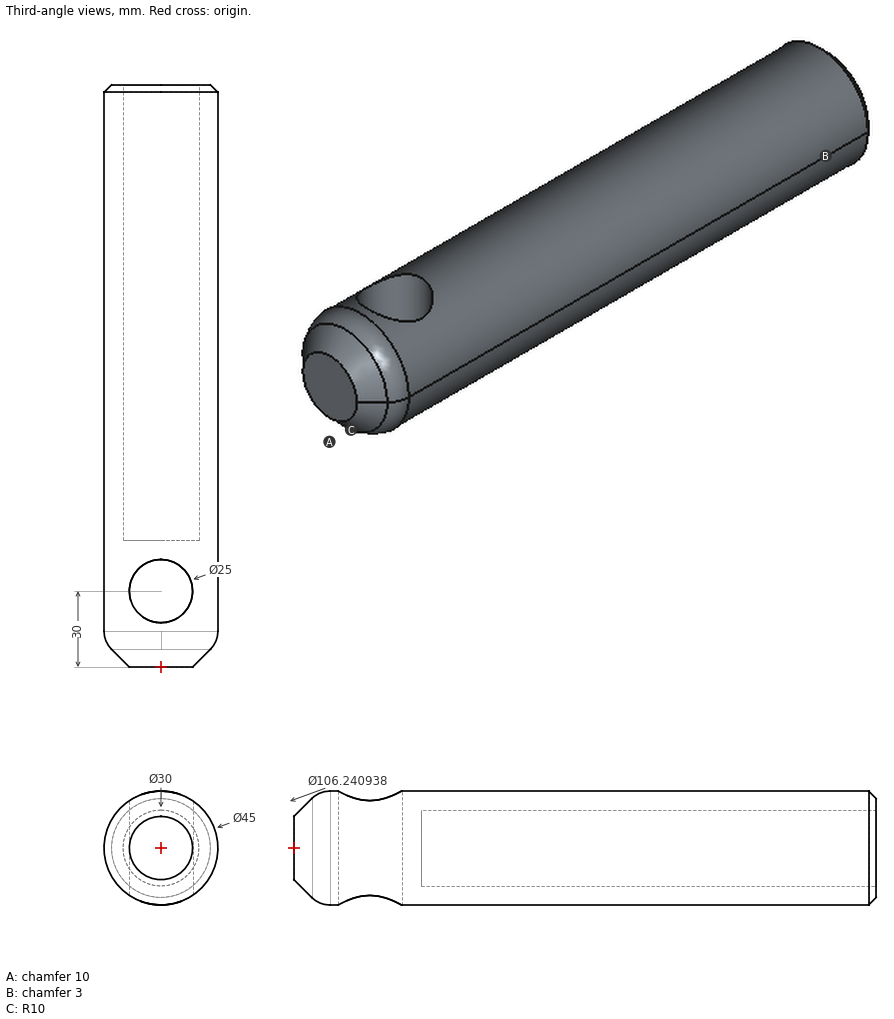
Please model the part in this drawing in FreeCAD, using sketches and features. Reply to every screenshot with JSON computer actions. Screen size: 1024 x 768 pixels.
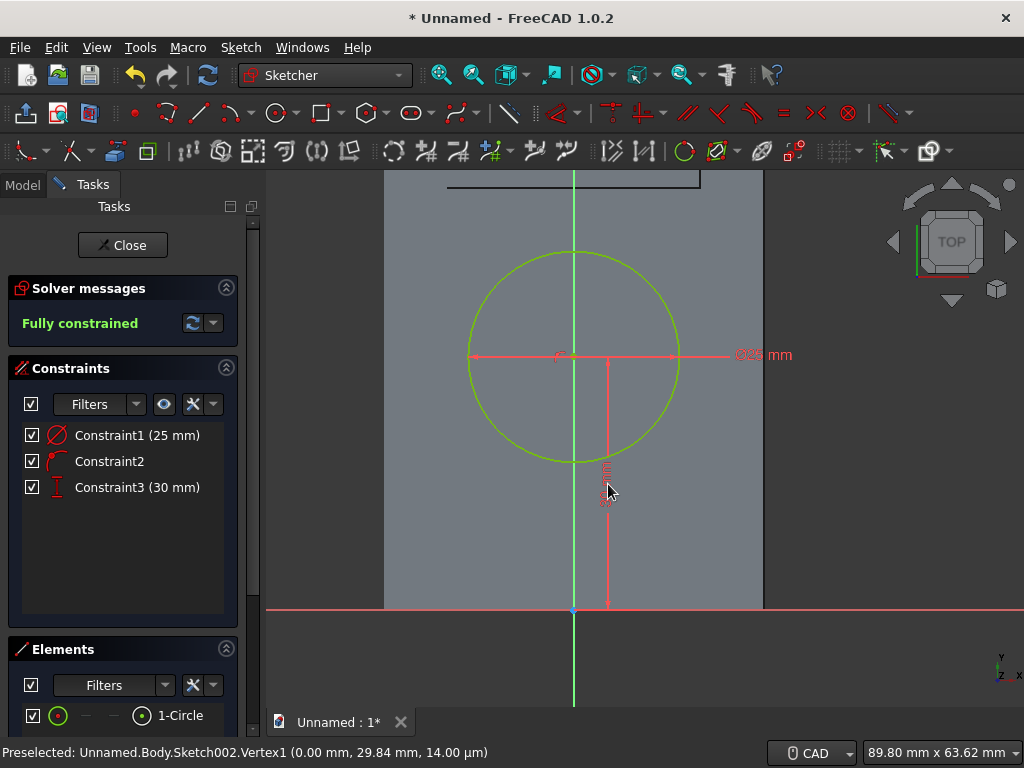
{"action": "left_click", "coordinate": [123, 245]}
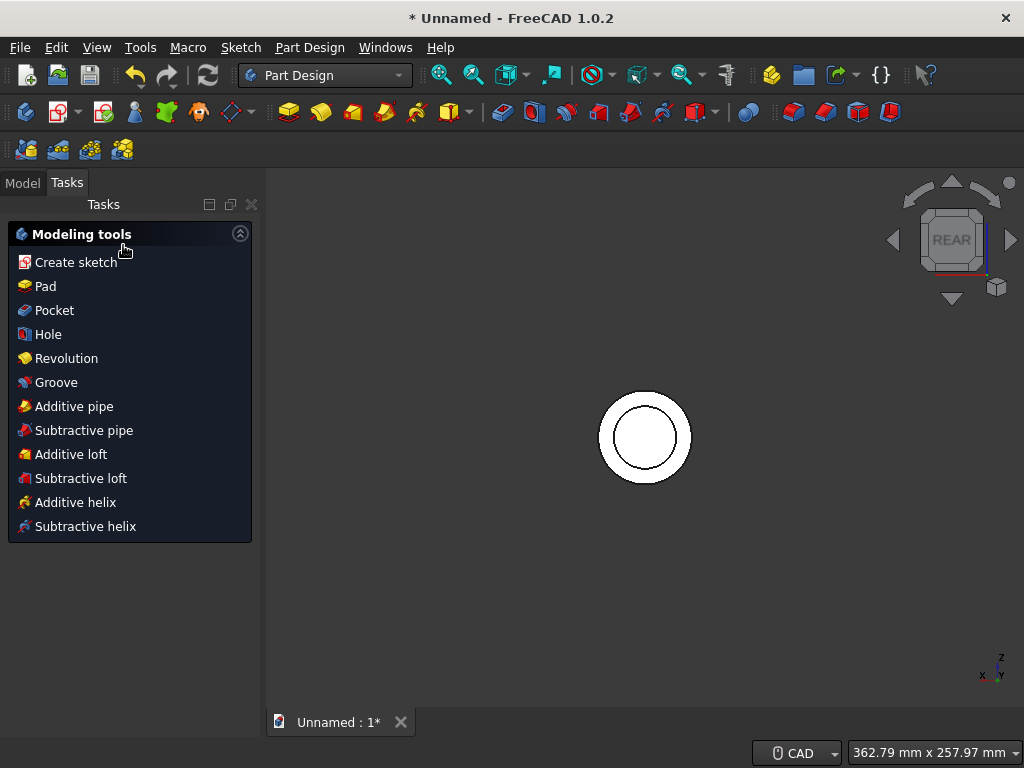
{"action": "left_click", "coordinate": [504, 112]}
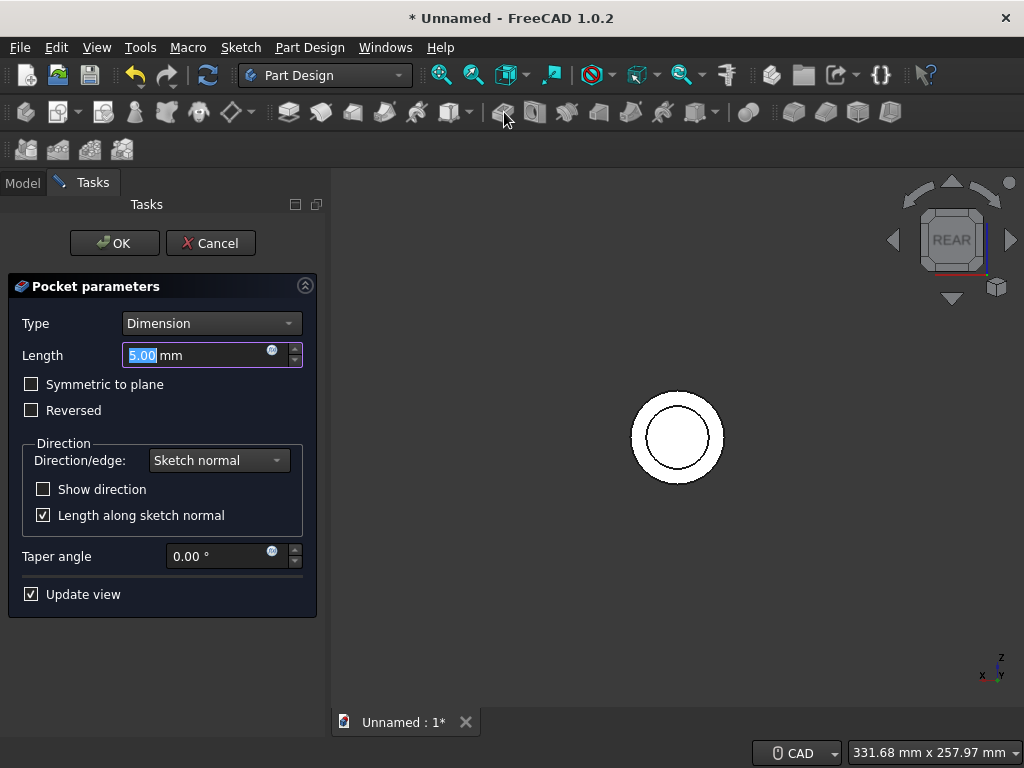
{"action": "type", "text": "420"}
{"action": "key", "text": "Tab"}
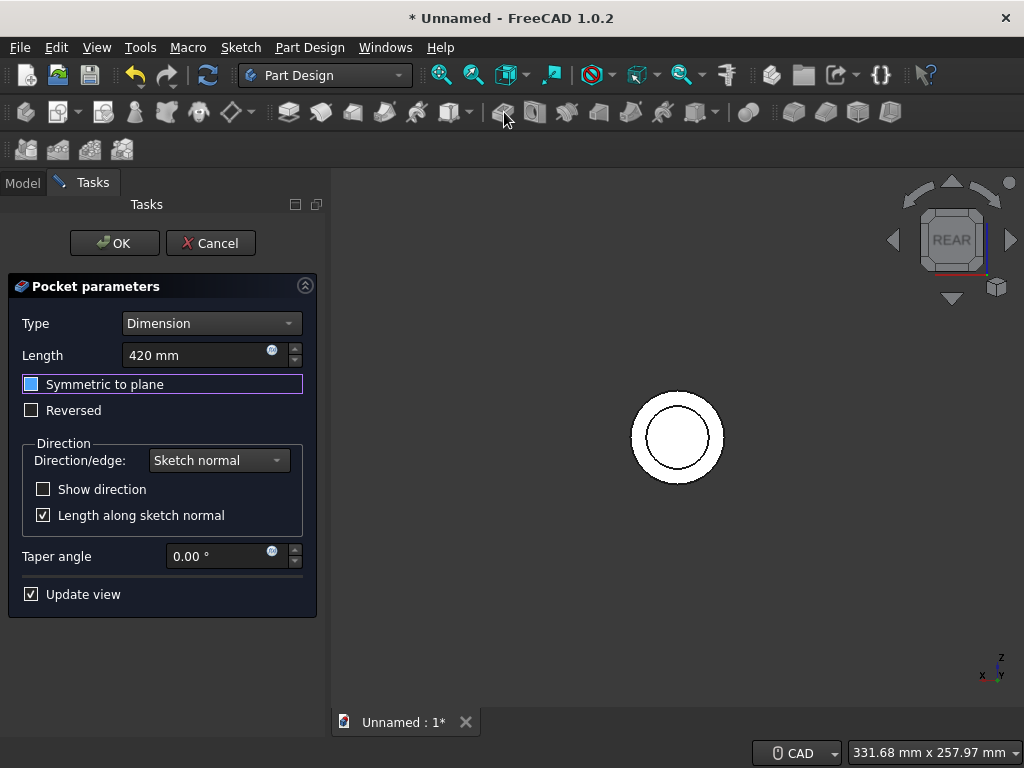
{"action": "left_click", "coordinate": [30, 384]}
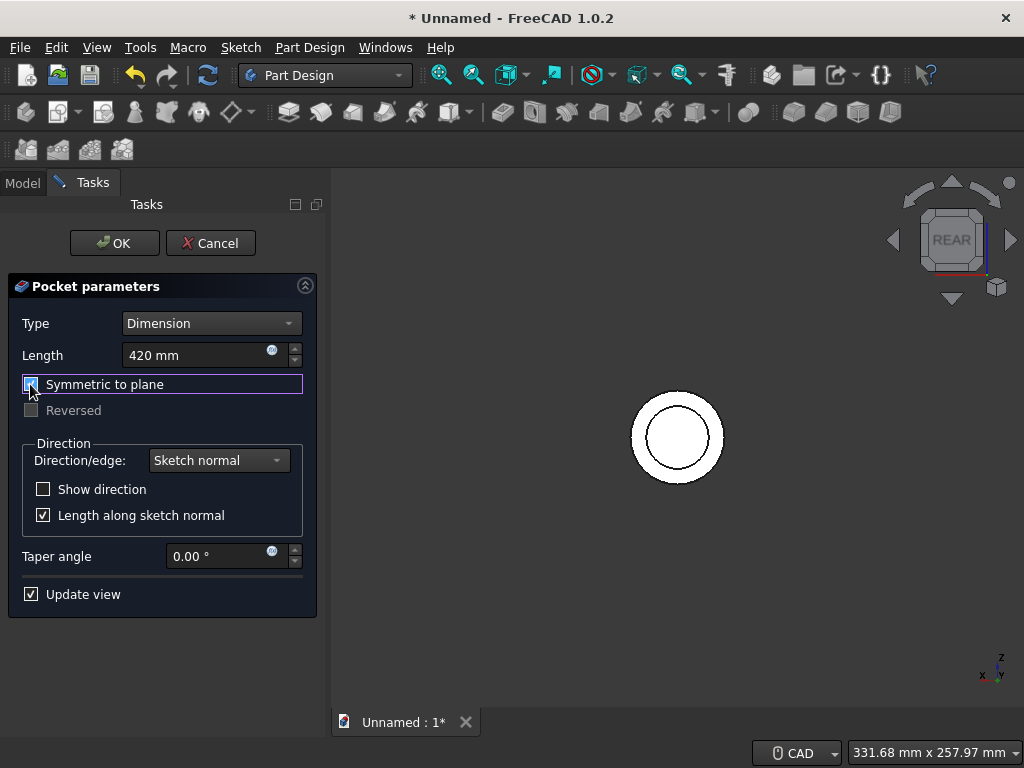
{"action": "left_click", "coordinate": [115, 243]}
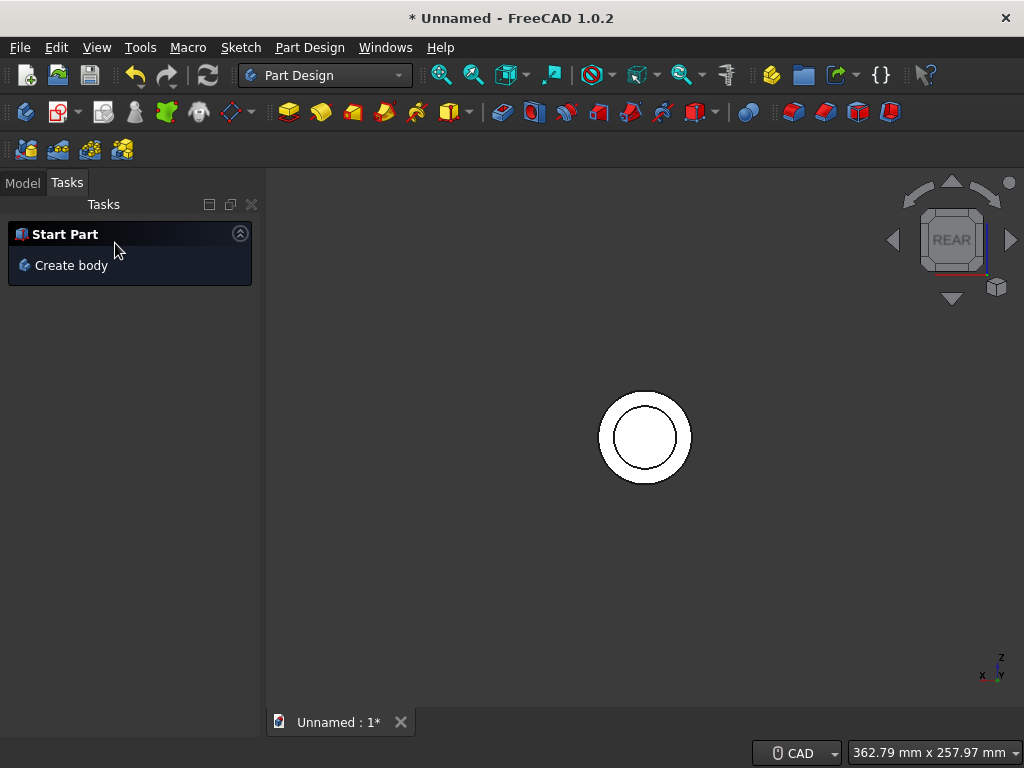
{"action": "left_click", "coordinate": [442, 76]}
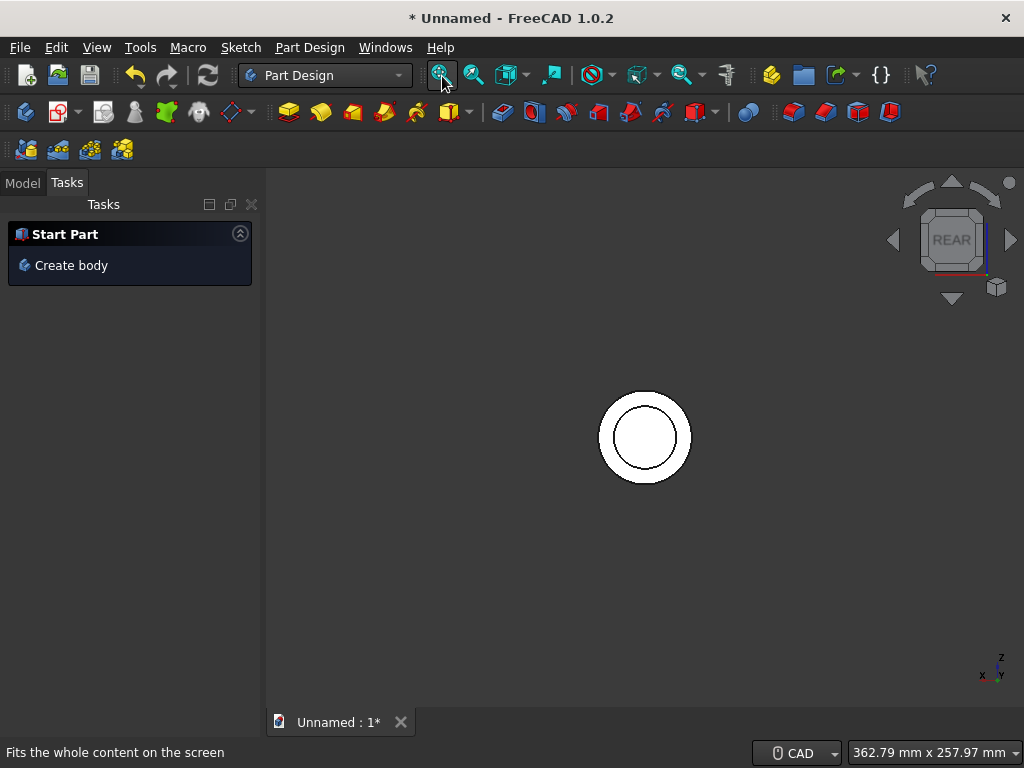
{"action": "left_click", "coordinate": [605, 436]}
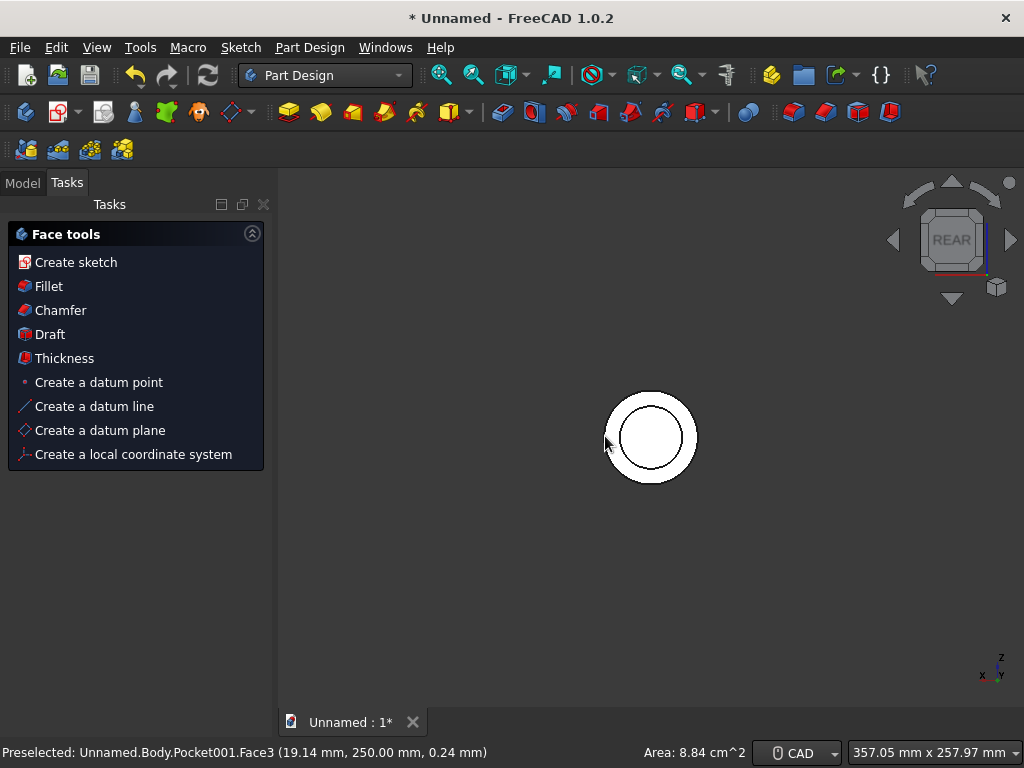
{"action": "left_click", "coordinate": [58, 112]}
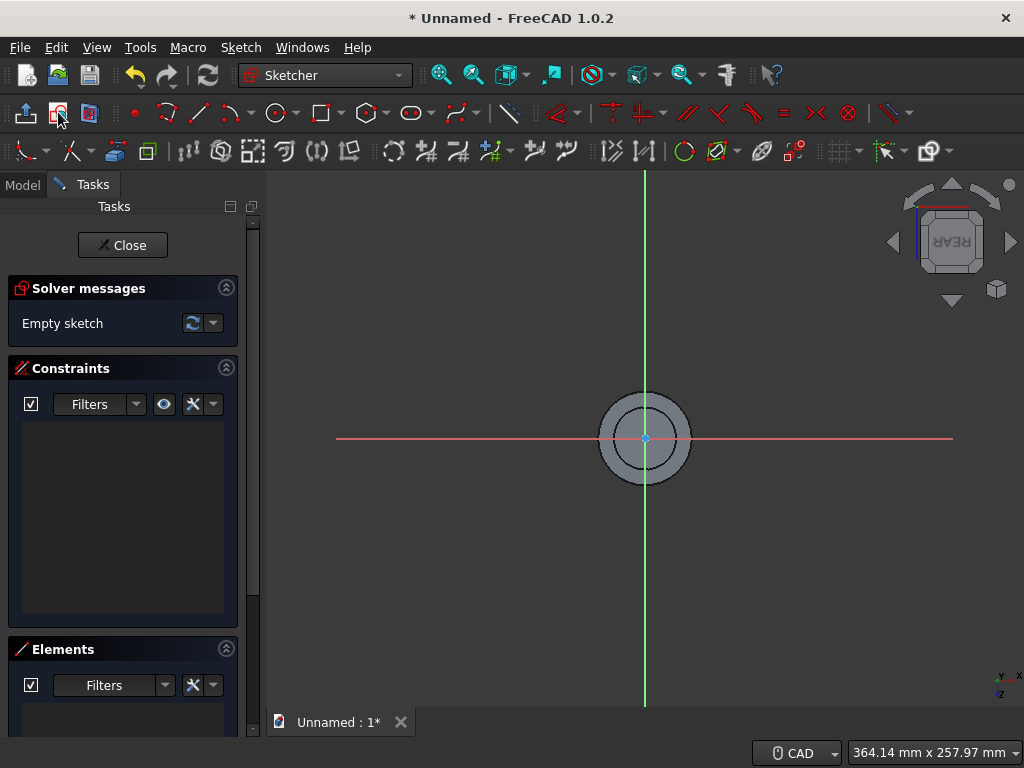
{"action": "scroll", "coordinate": [784, 438], "scroll_direction": "up", "scroll_amount": 2}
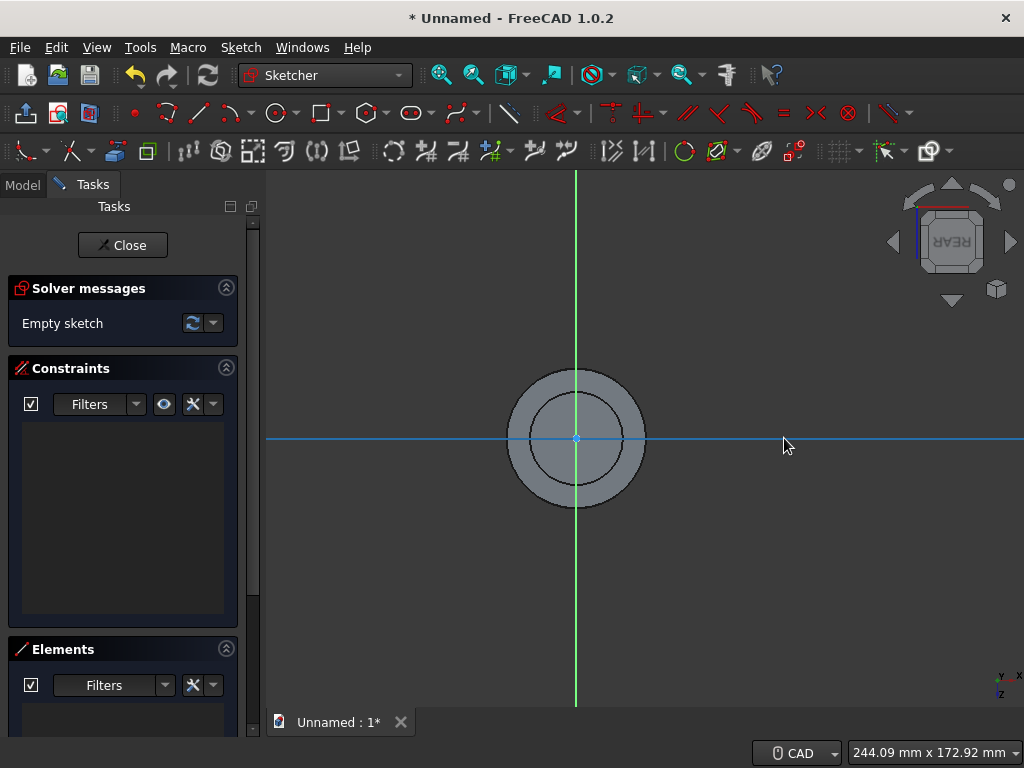
{"action": "left_click", "coordinate": [276, 114]}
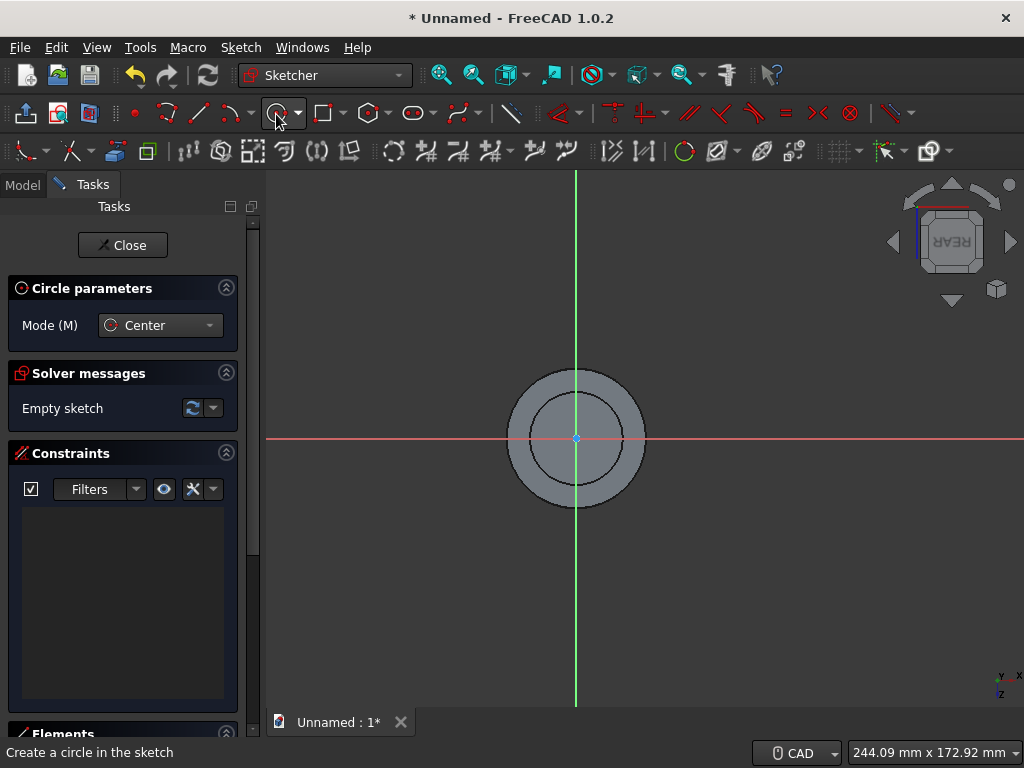
{"action": "left_click", "coordinate": [576, 438]}
{"action": "mouse_move", "coordinate": [693, 322]}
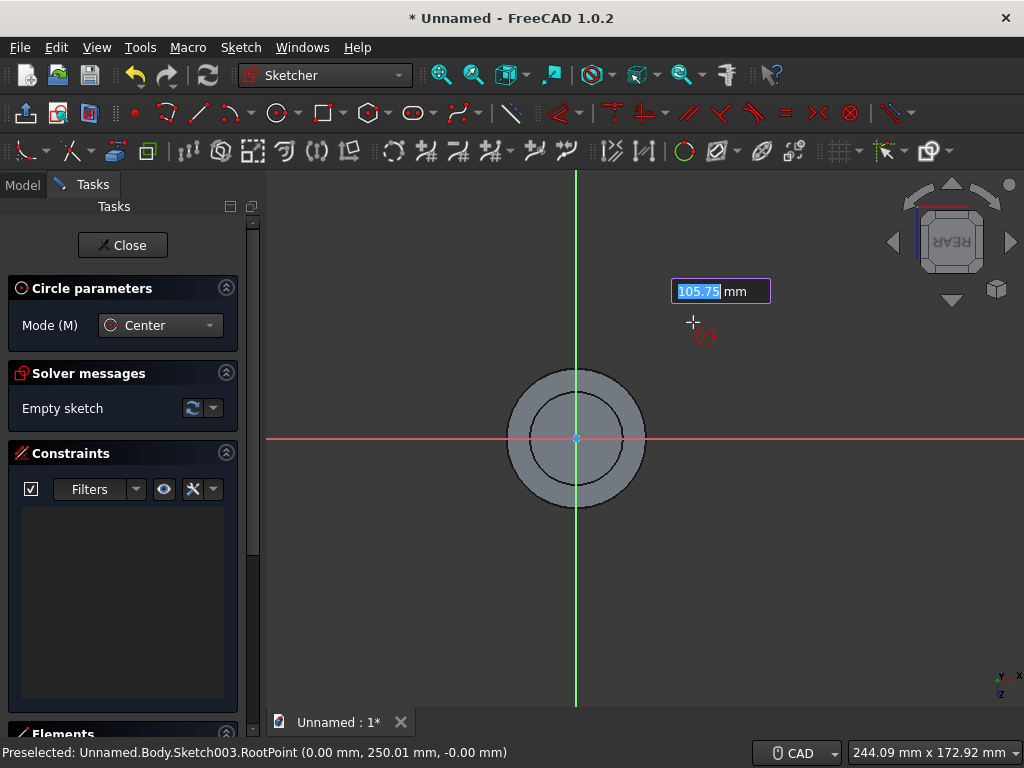
{"action": "type", "text": "106.240938"}
{"action": "key", "text": "Return"}
{"action": "key", "text": "Escape"}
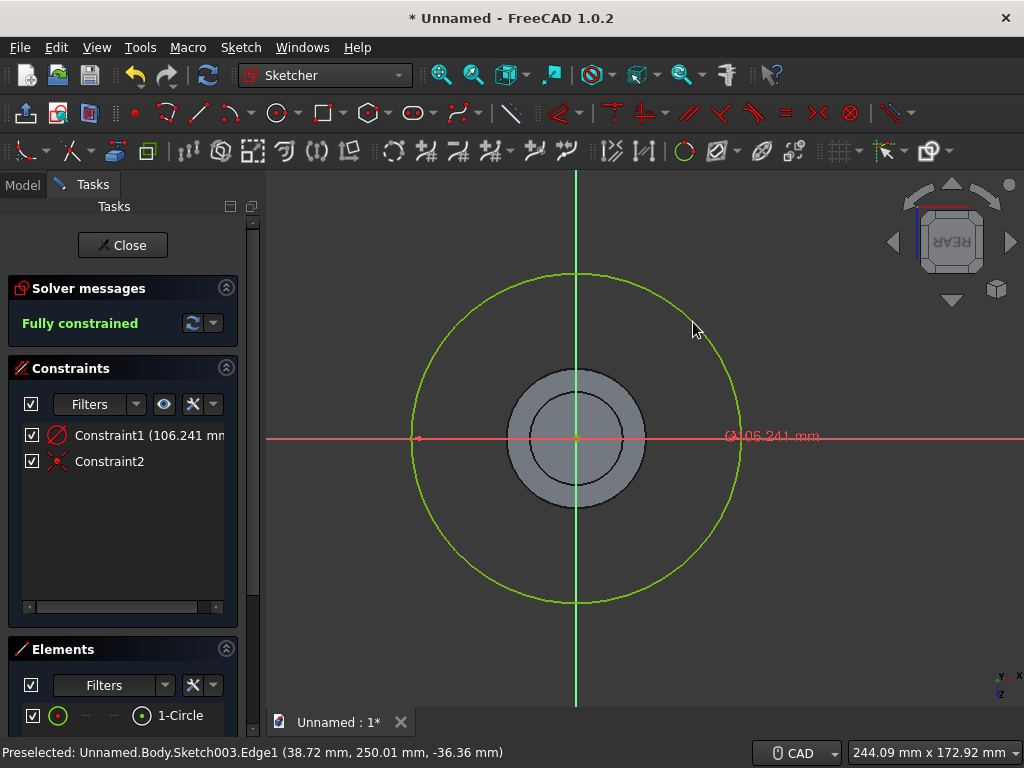
{"action": "left_click", "coordinate": [123, 245]}